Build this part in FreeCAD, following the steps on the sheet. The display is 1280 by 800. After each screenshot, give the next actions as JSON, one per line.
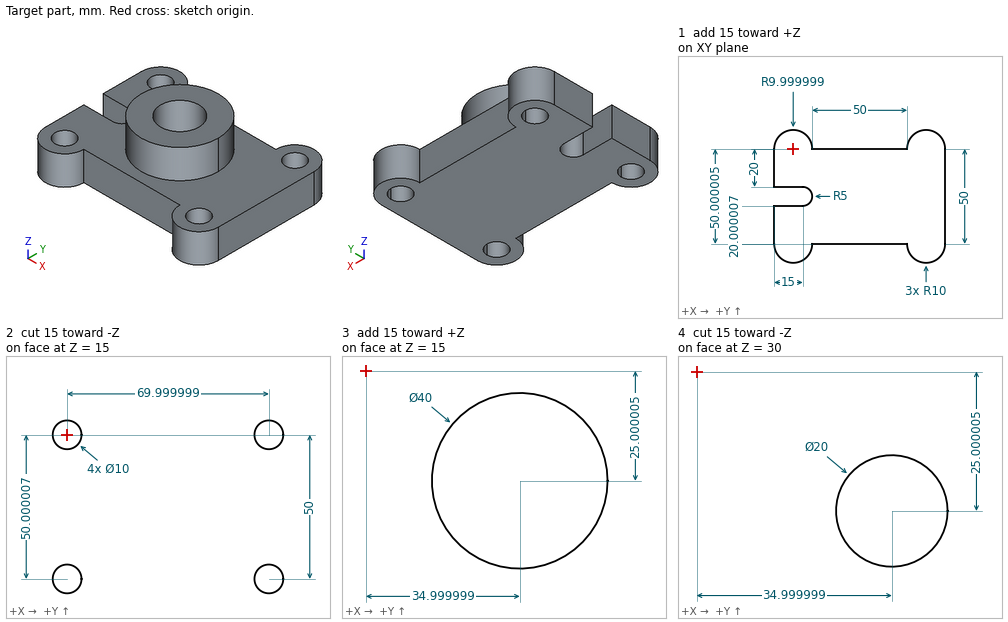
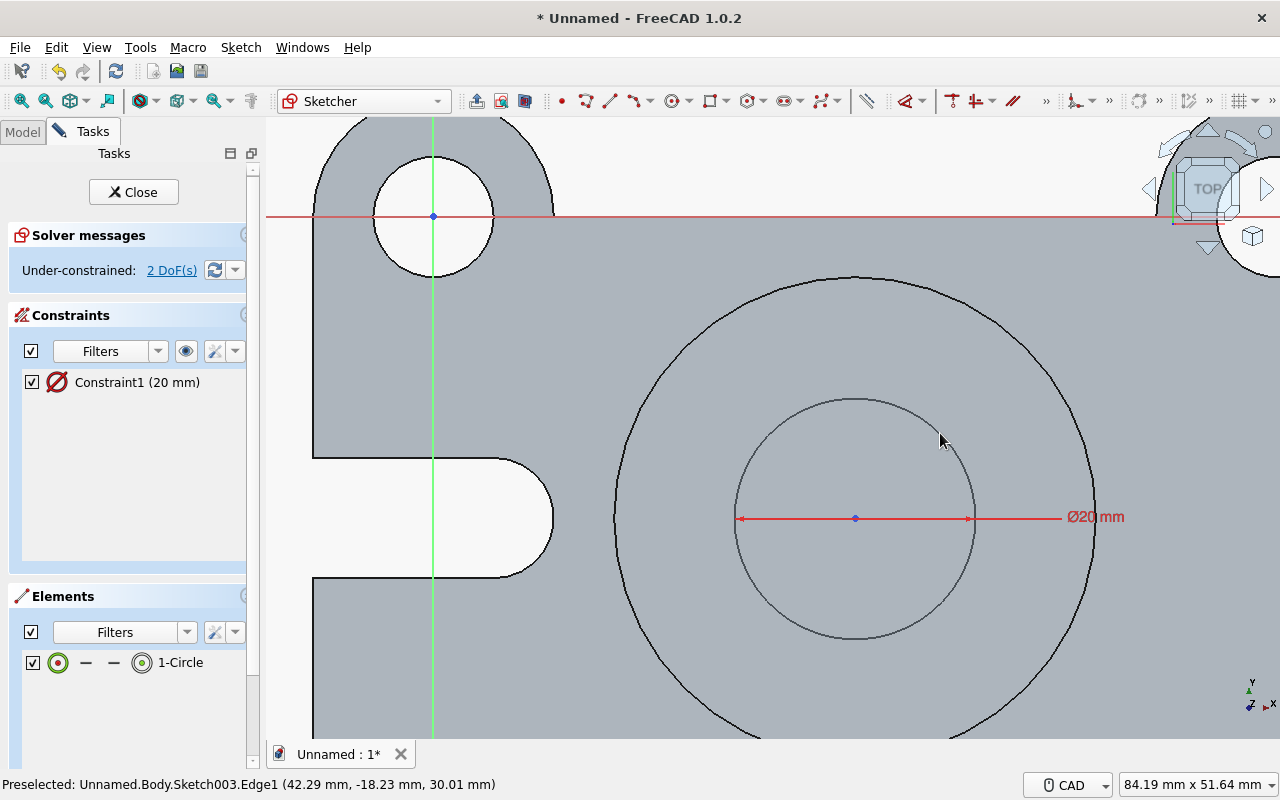
{"action": "left_click", "coordinate": [906, 102]}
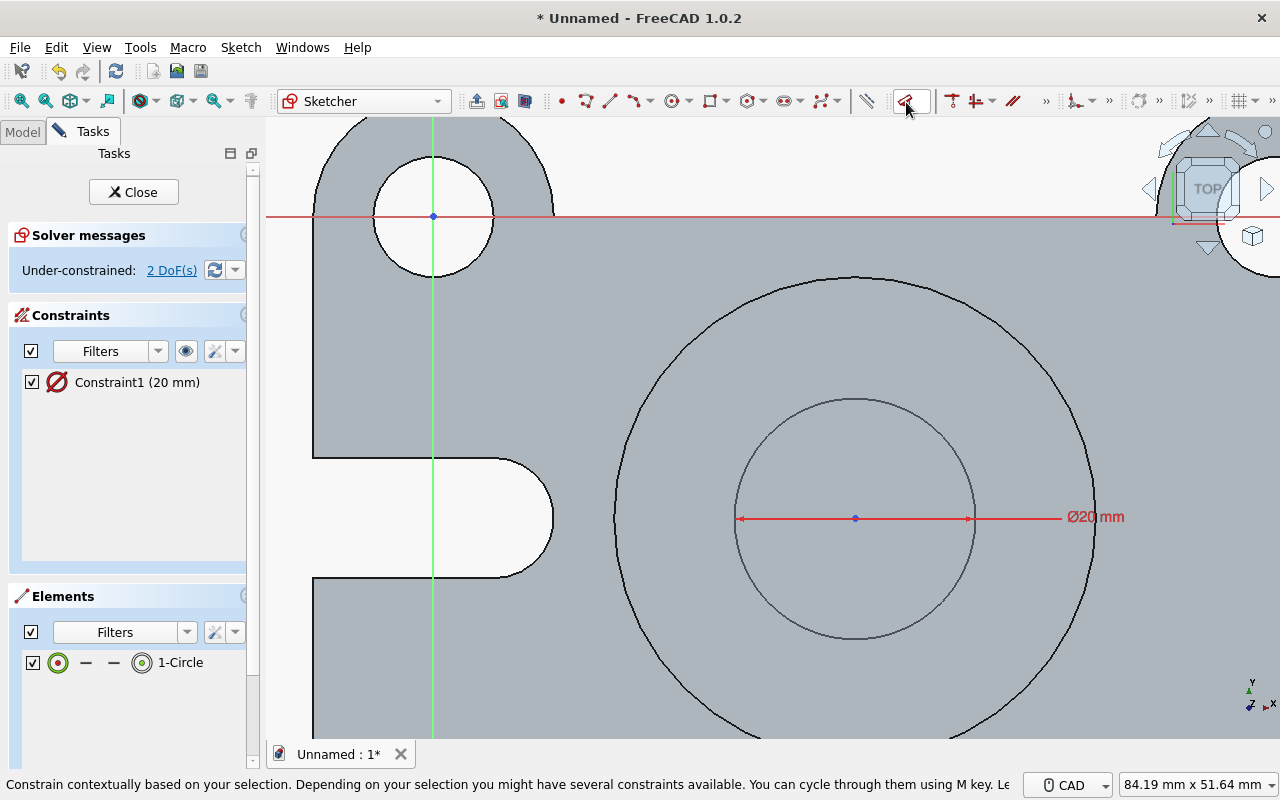
{"action": "left_click", "coordinate": [855, 519]}
{"action": "left_click", "coordinate": [644, 183]}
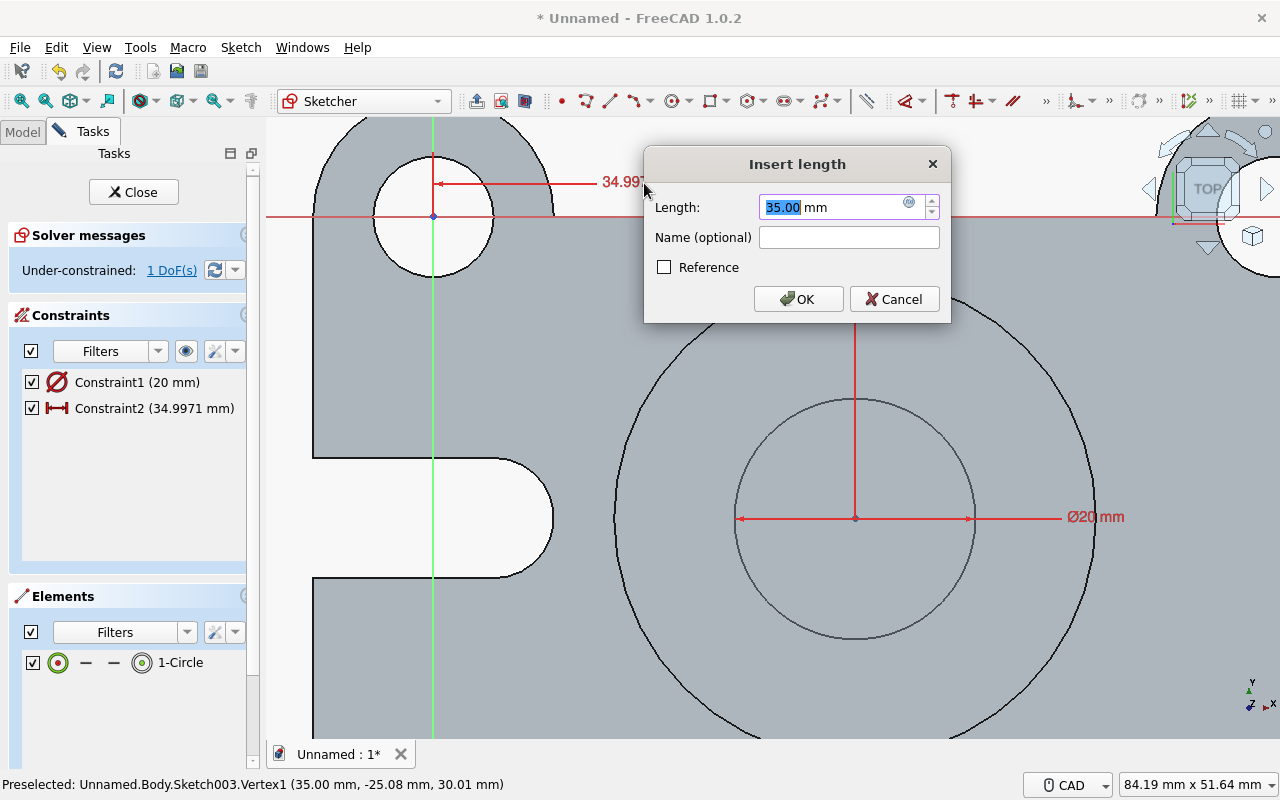
{"action": "type", "text": "34.999999"}
{"action": "key", "text": "Return"}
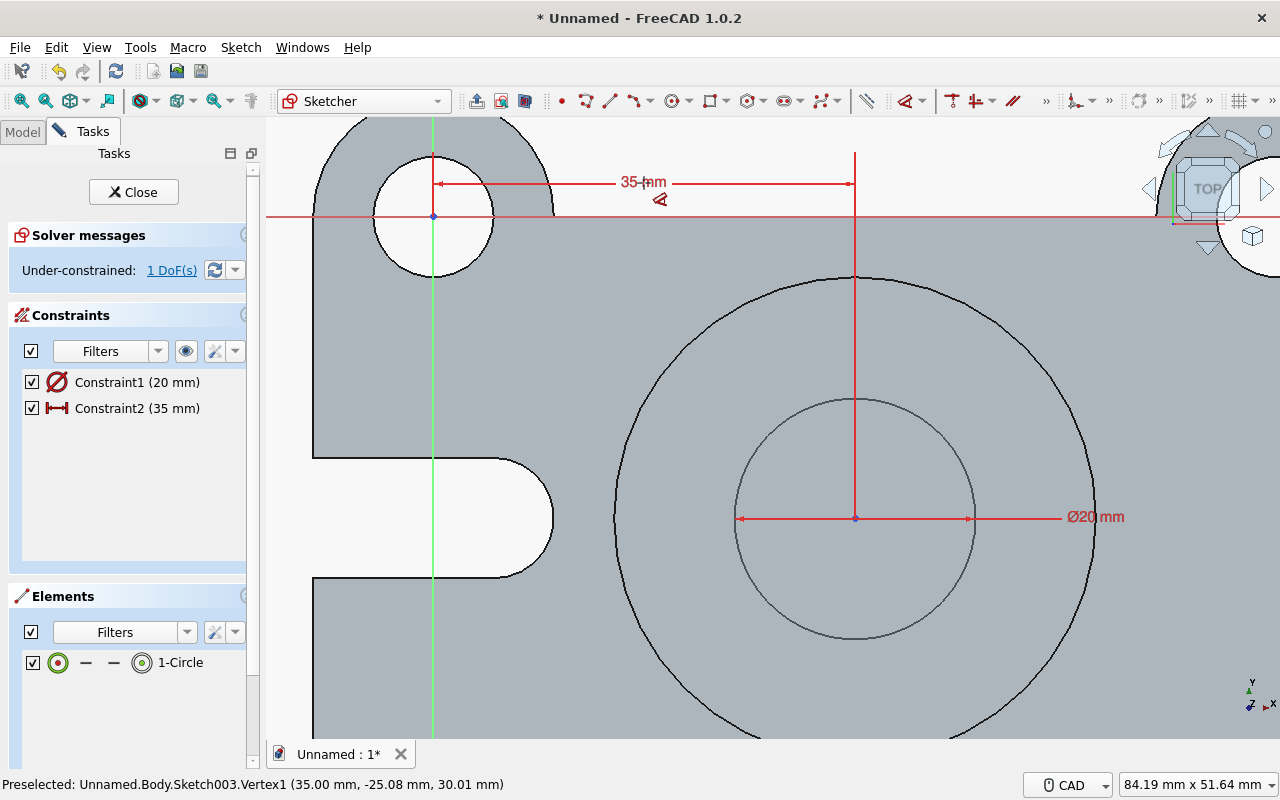
{"action": "left_click", "coordinate": [855, 519]}
{"action": "left_click", "coordinate": [399, 368]}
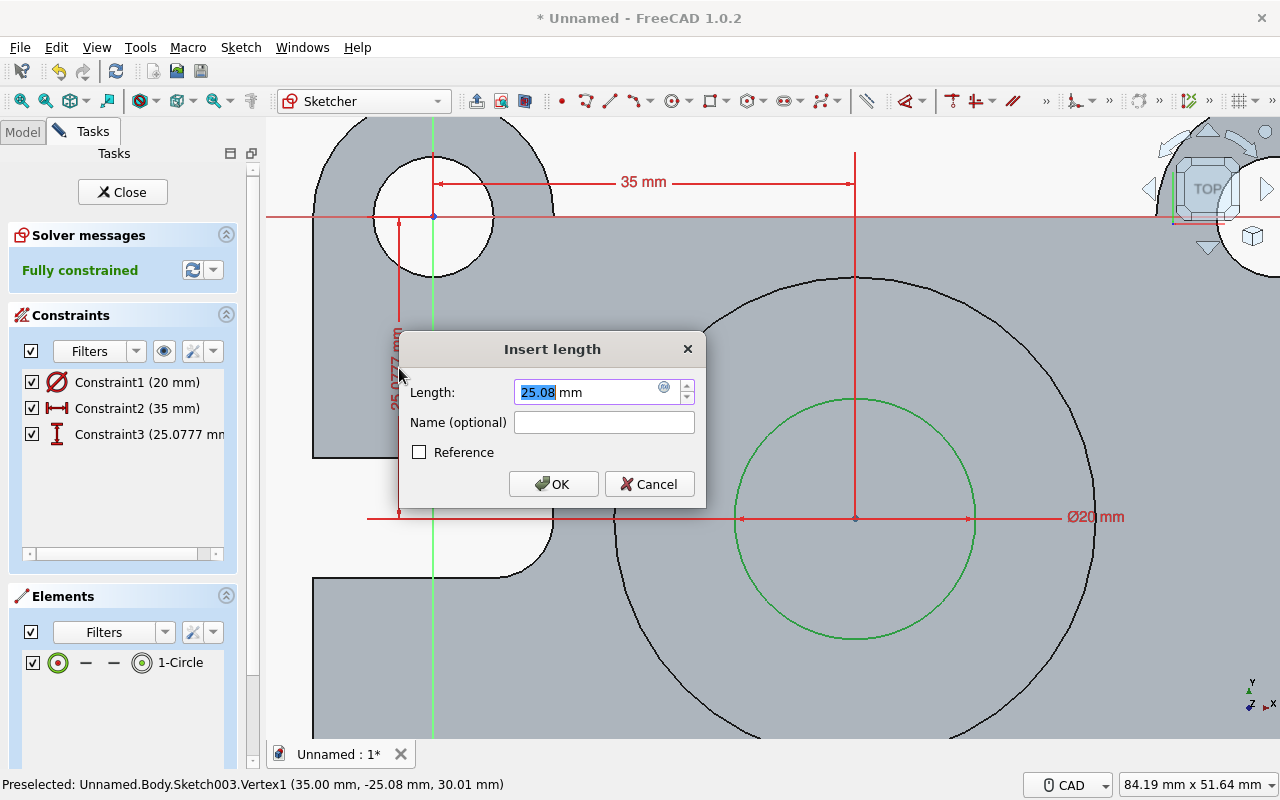
{"action": "type", "text": "25.000005"}
{"action": "key", "text": "Return"}
{"action": "key", "text": "Escape"}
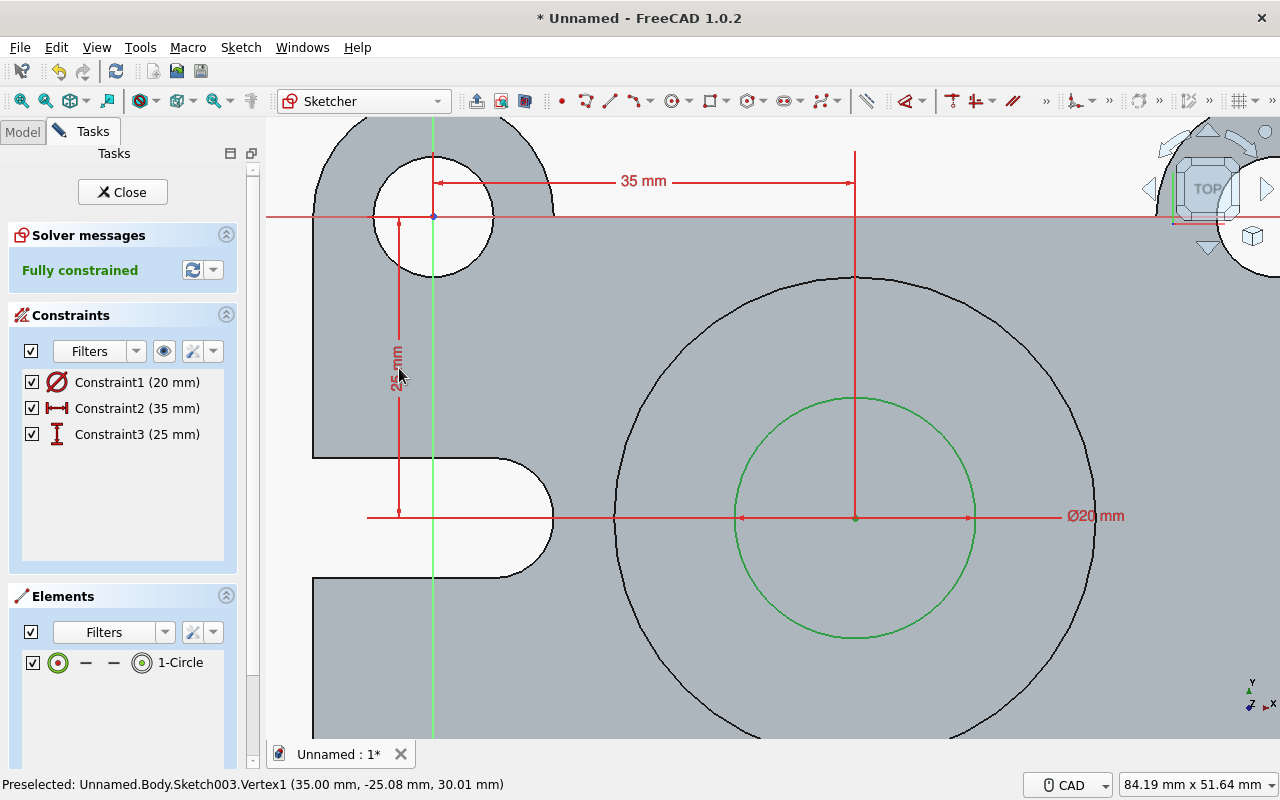
{"action": "left_click", "coordinate": [123, 192]}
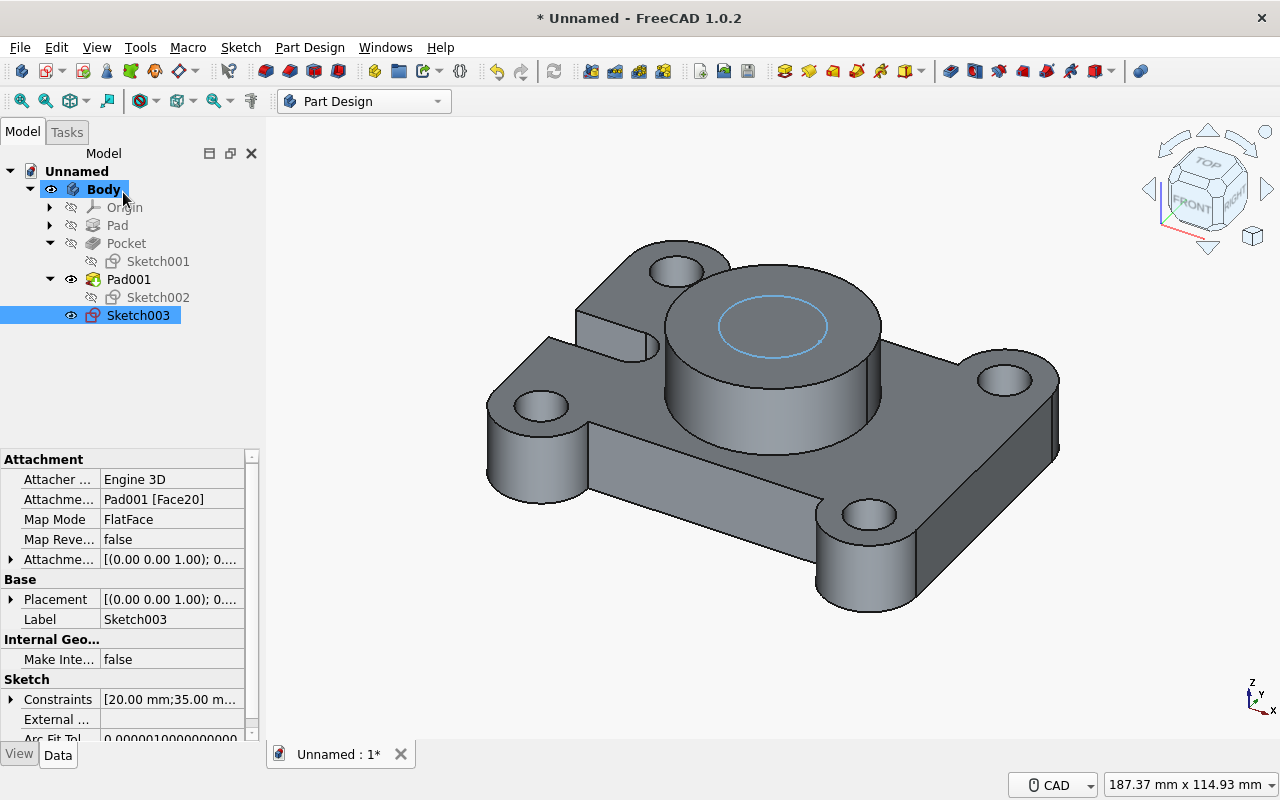
{"action": "left_click", "coordinate": [952, 72]}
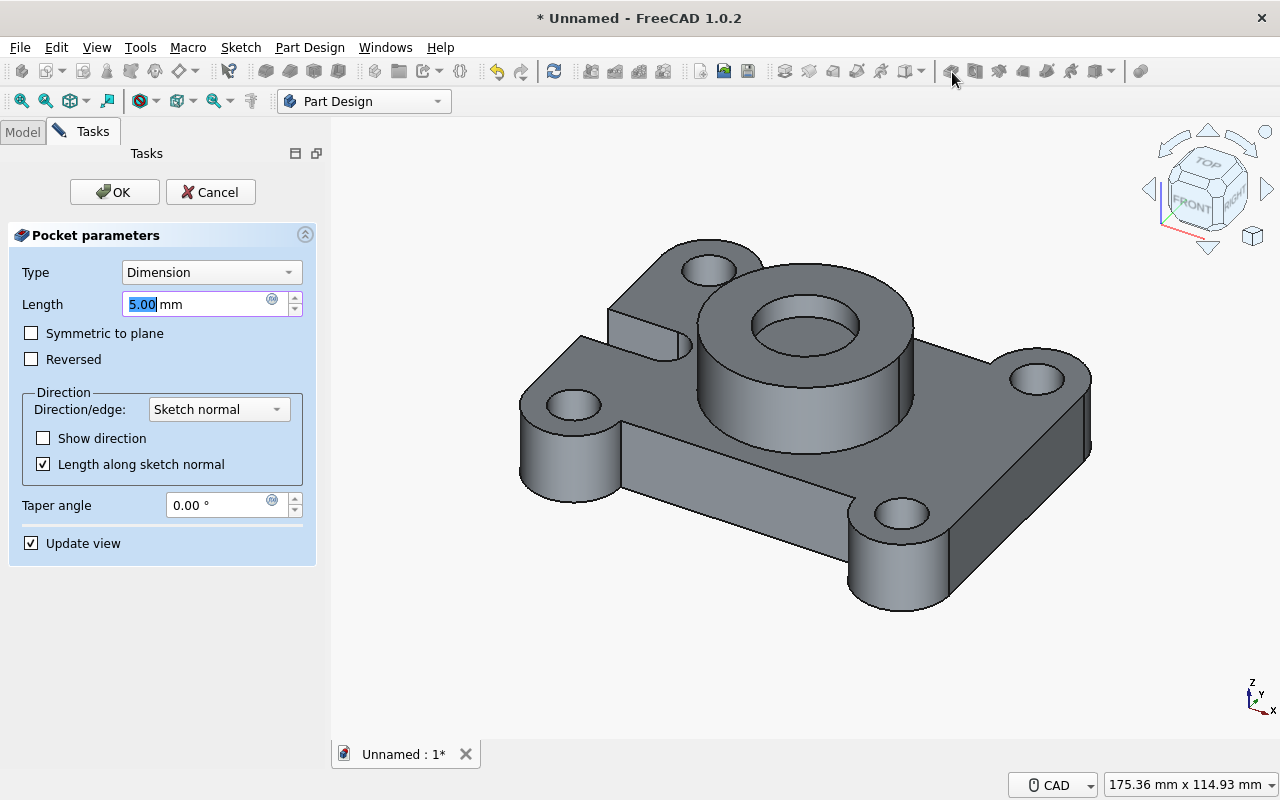
{"action": "type", "text": "15"}
{"action": "key", "text": "Tab"}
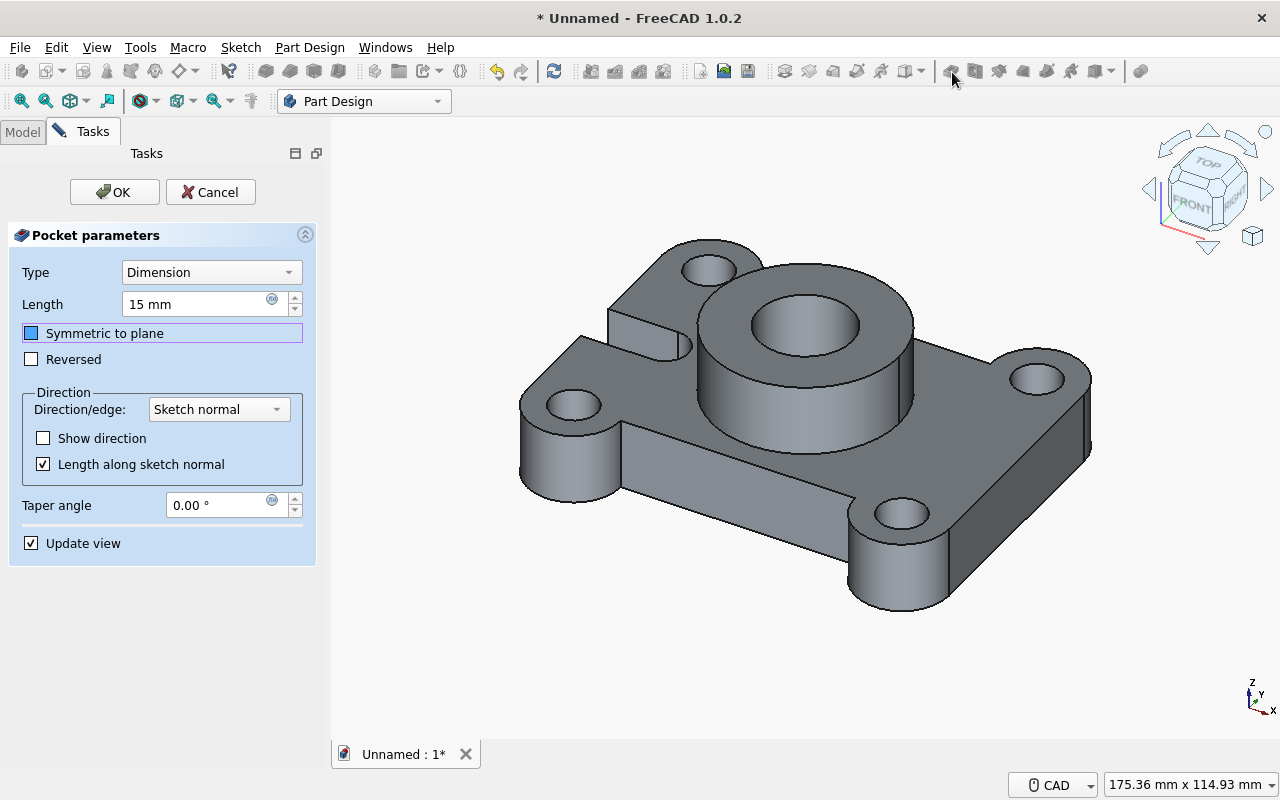
{"action": "left_click", "coordinate": [115, 192]}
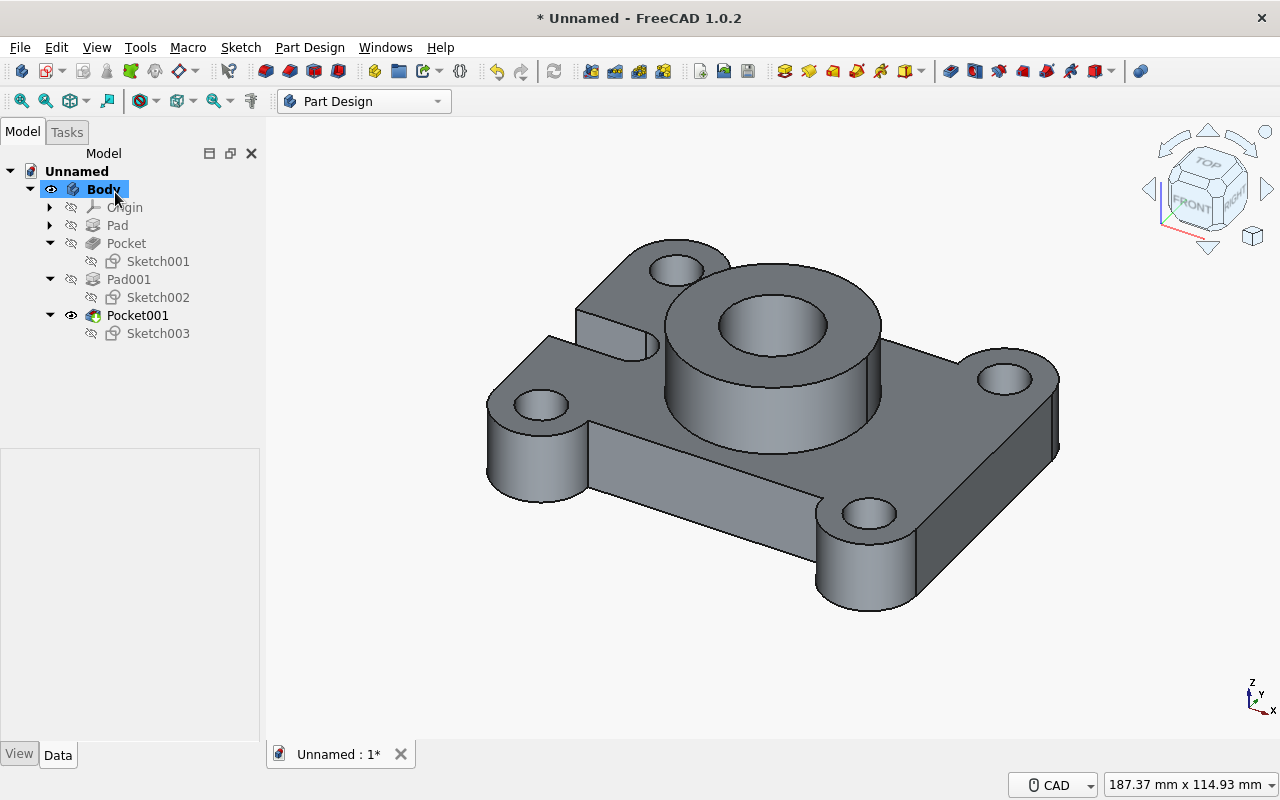
{"action": "key", "text": "0"}